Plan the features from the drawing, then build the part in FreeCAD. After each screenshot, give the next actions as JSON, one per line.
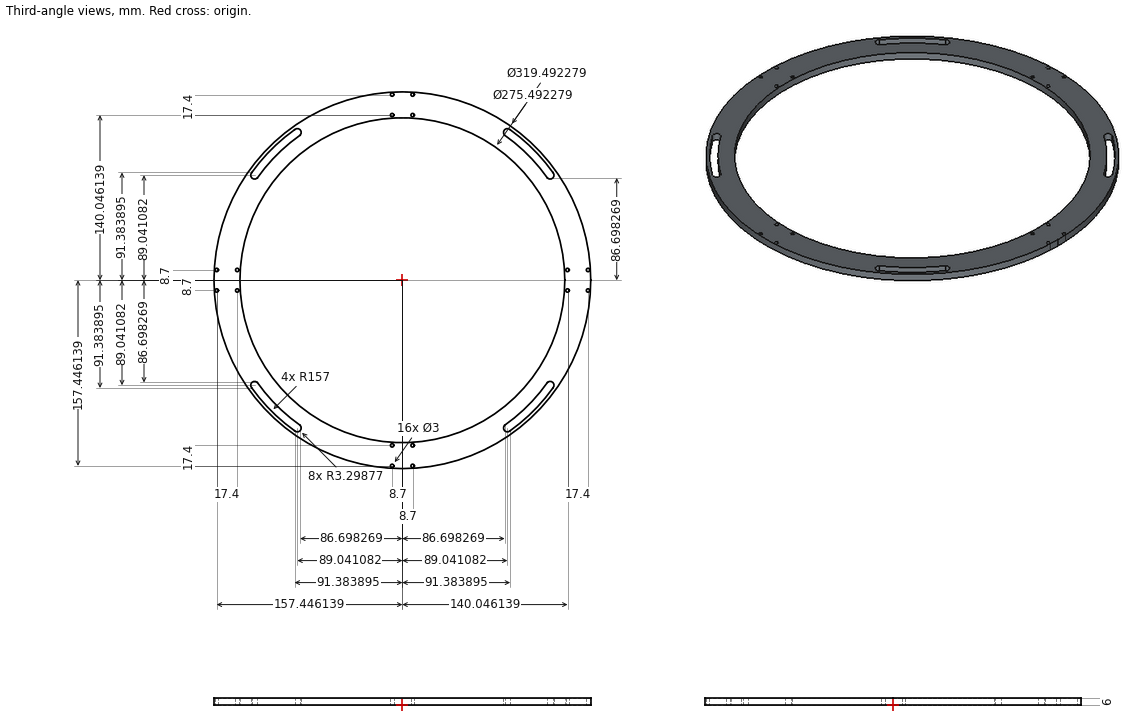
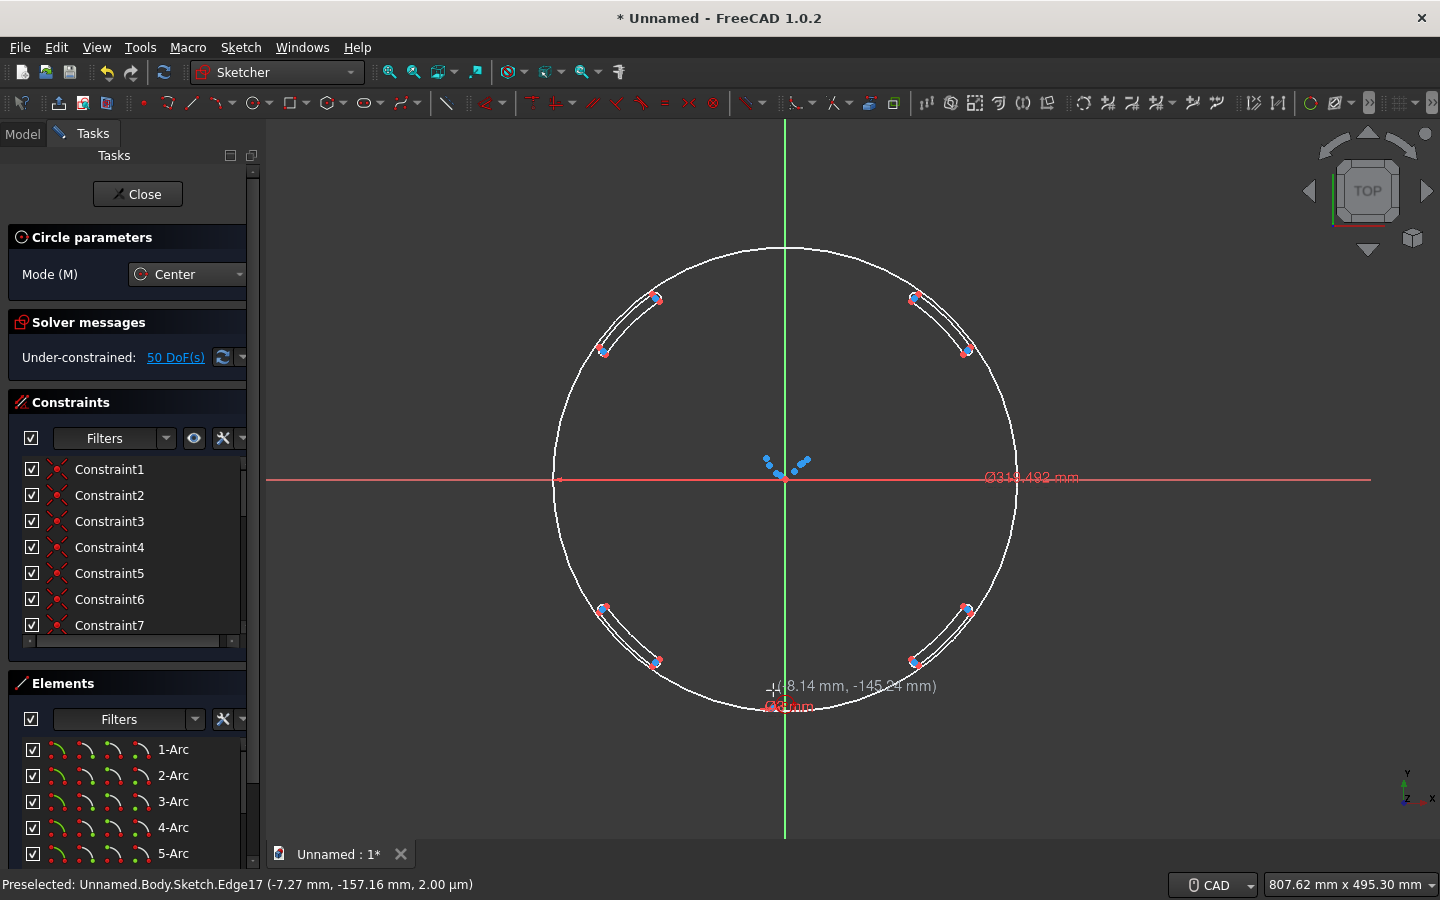
{"action": "scroll", "coordinate": [773, 683], "scroll_direction": "up", "scroll_amount": 2}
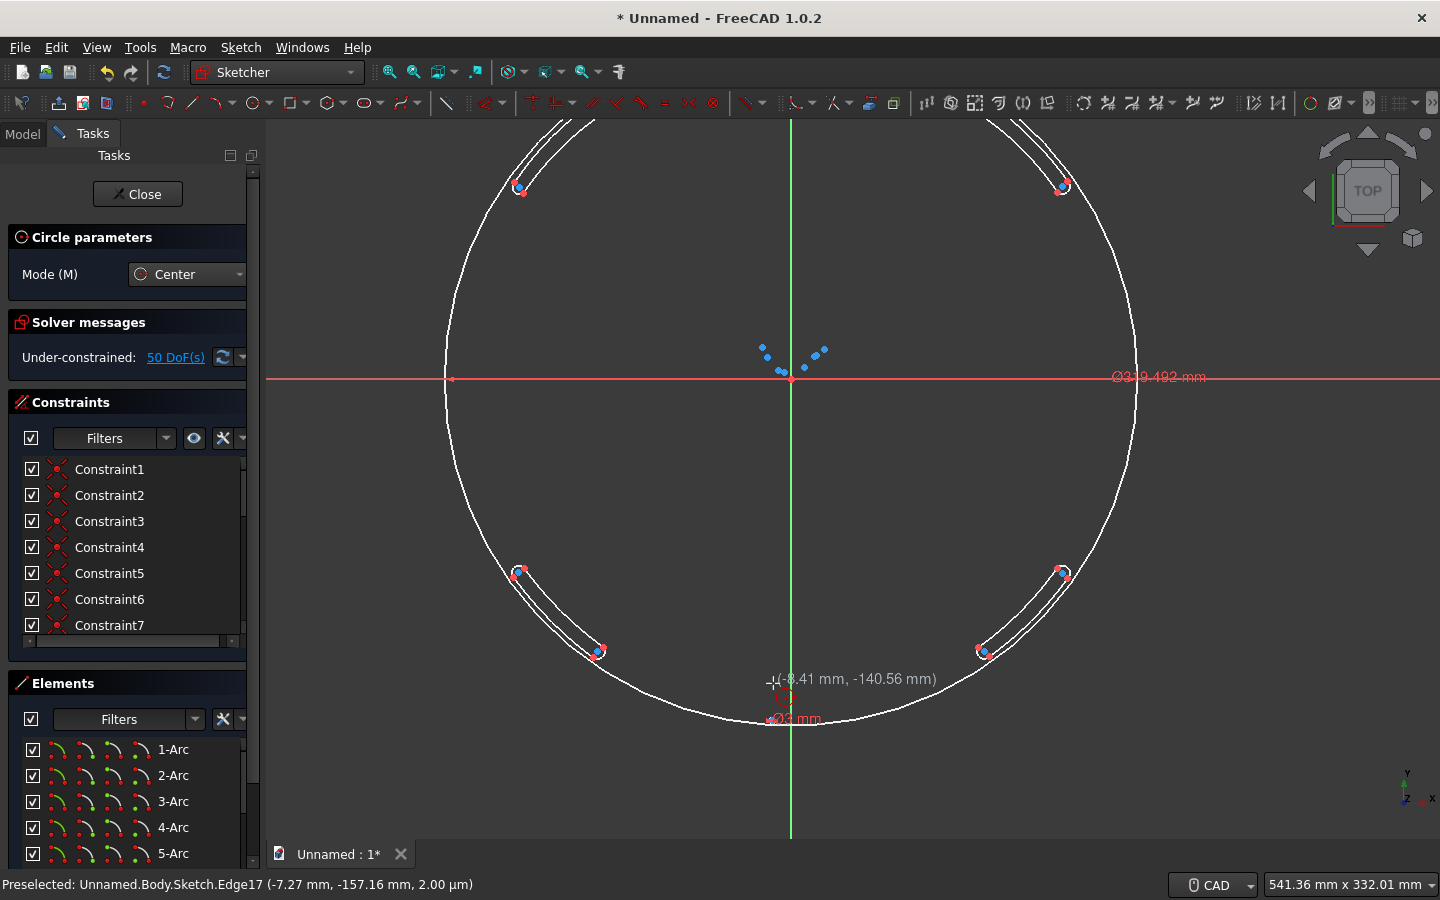
{"action": "left_click", "coordinate": [772, 683]}
{"action": "mouse_move", "coordinate": [774, 681]}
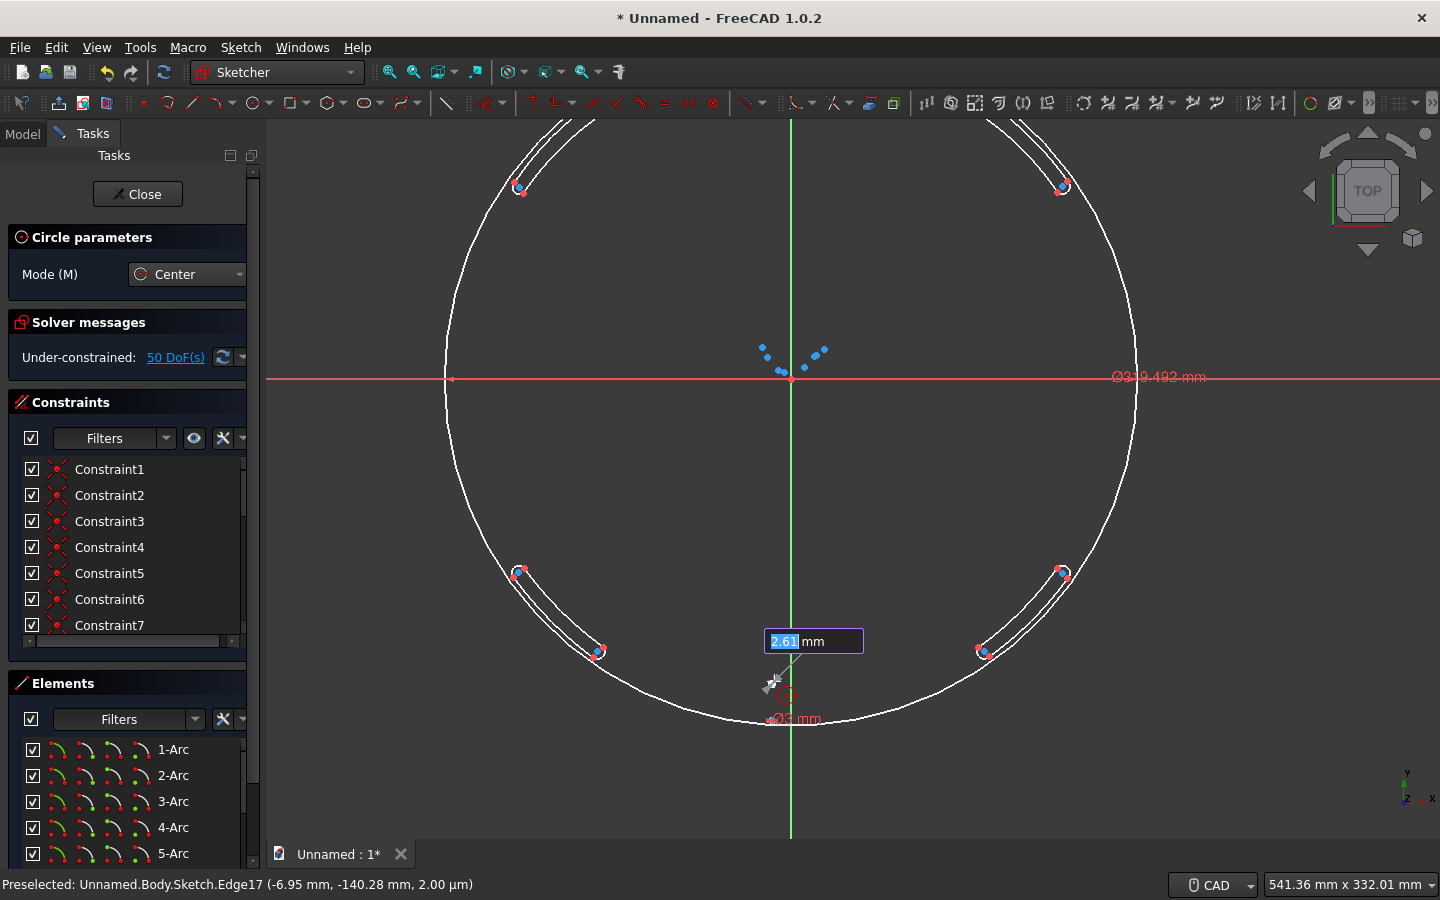
{"action": "type", "text": "3"}
{"action": "key", "text": "Return"}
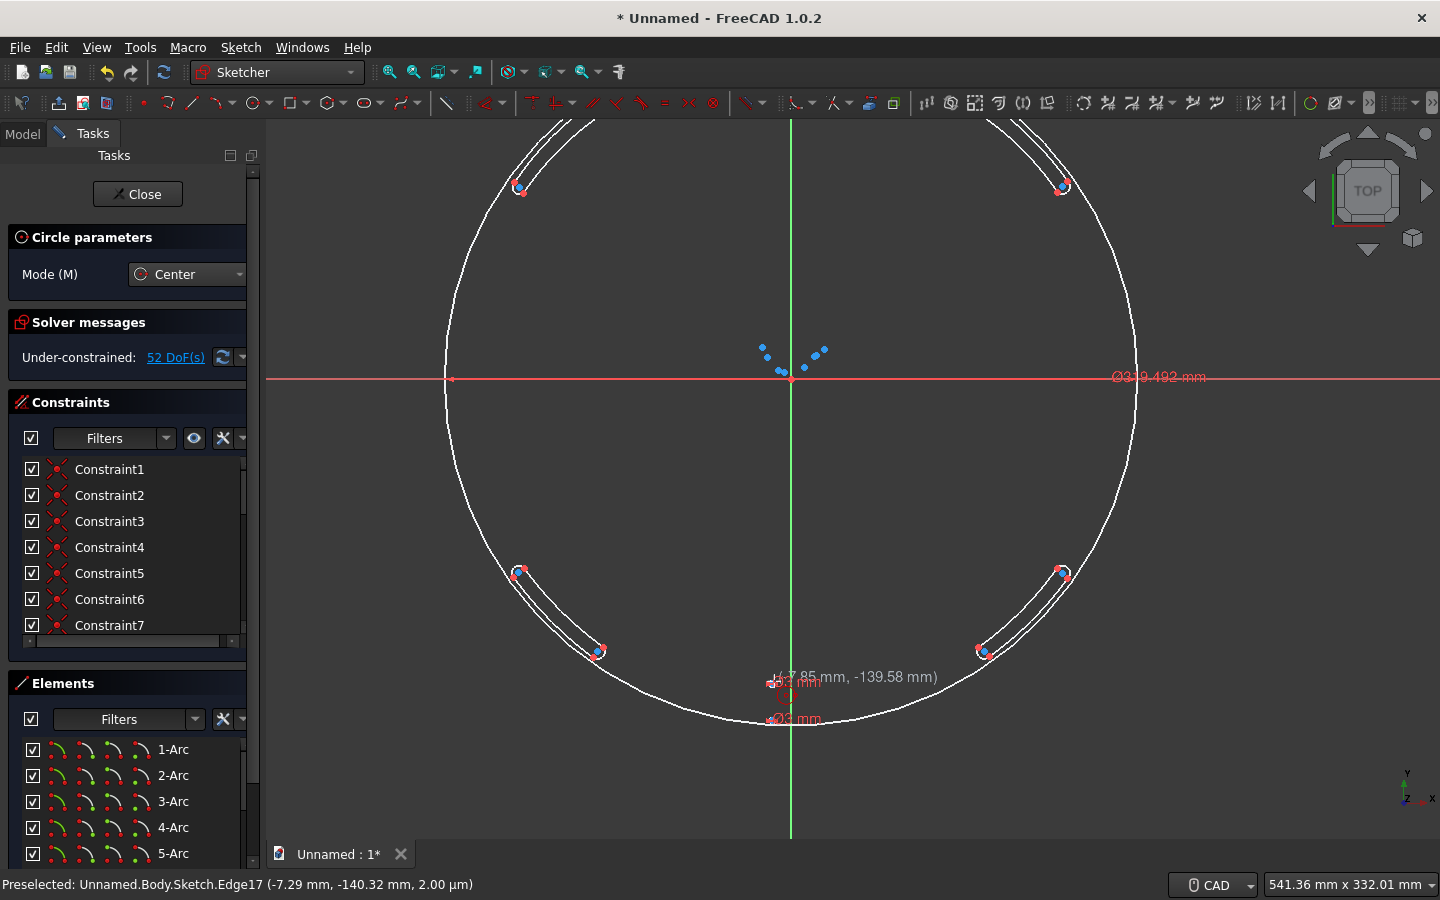
{"action": "scroll", "coordinate": [450, 398], "scroll_direction": "up", "scroll_amount": 10}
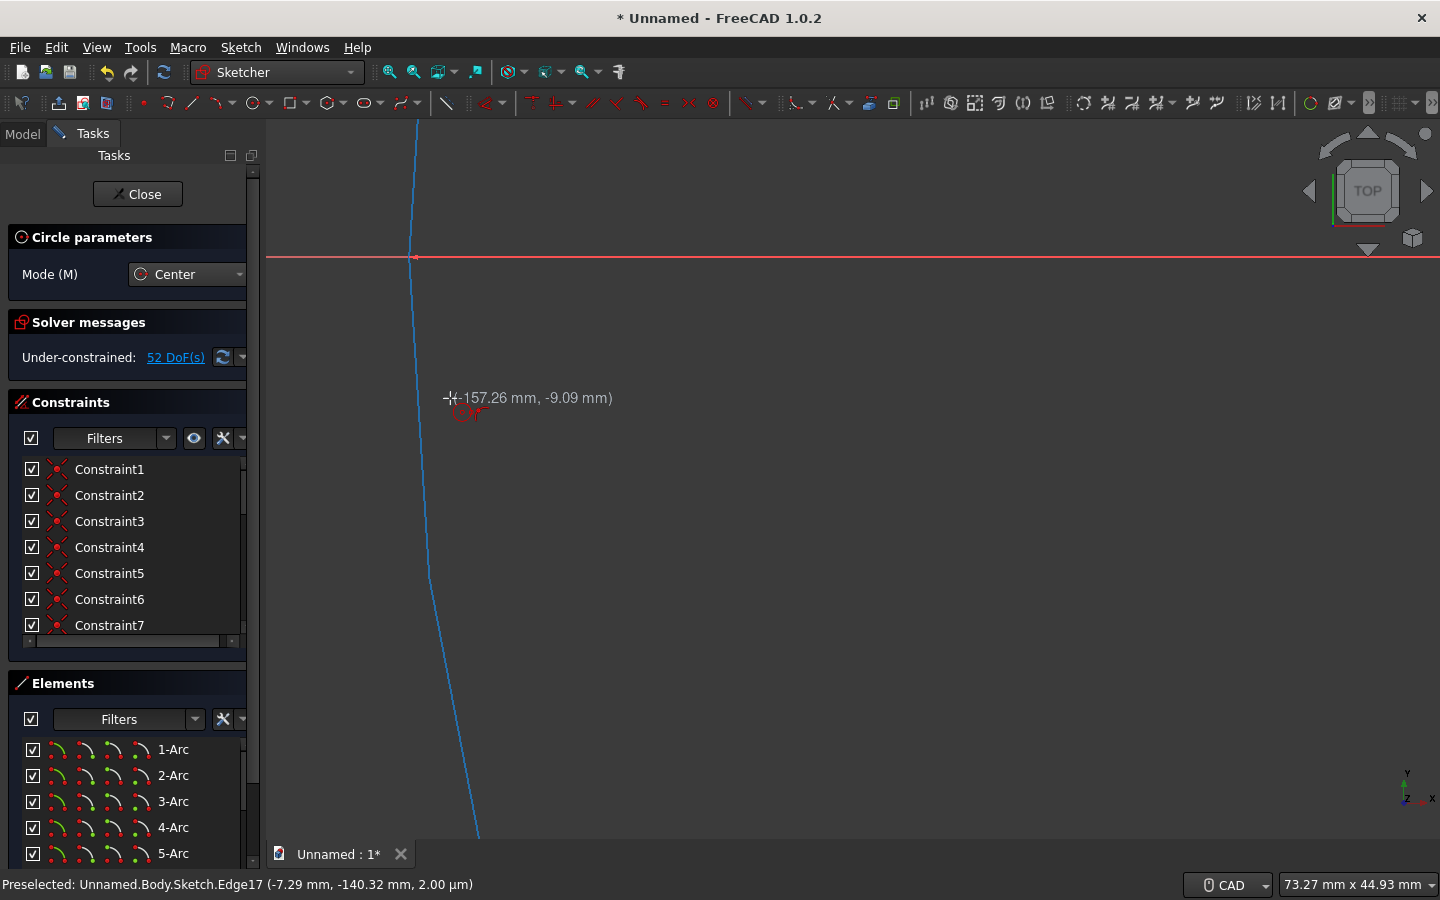
{"action": "left_click", "coordinate": [446, 397]}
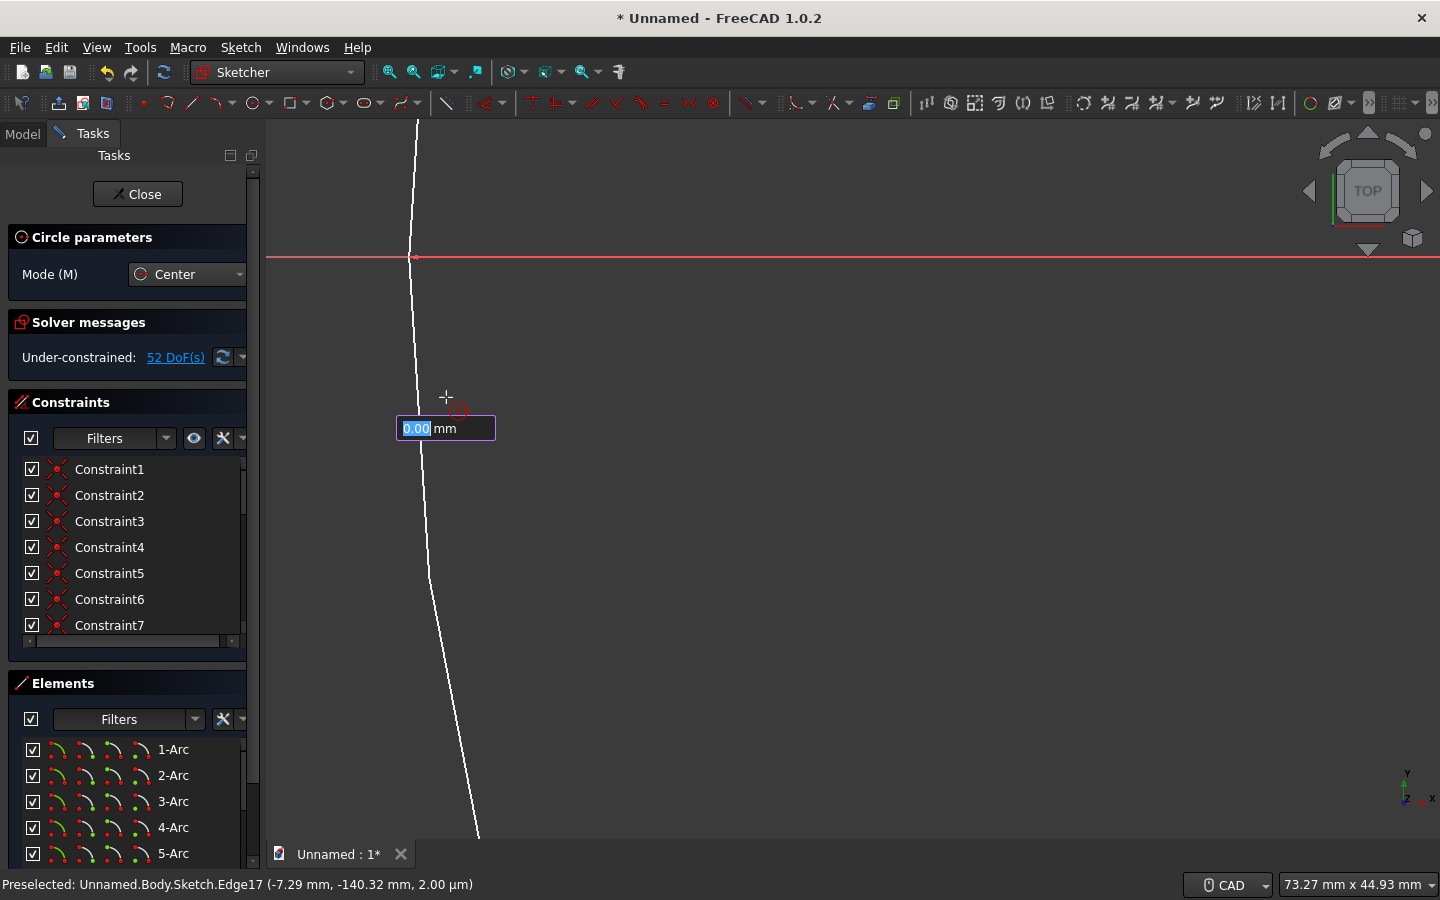
{"action": "scroll", "coordinate": [567, 501], "scroll_direction": "down", "scroll_amount": 12}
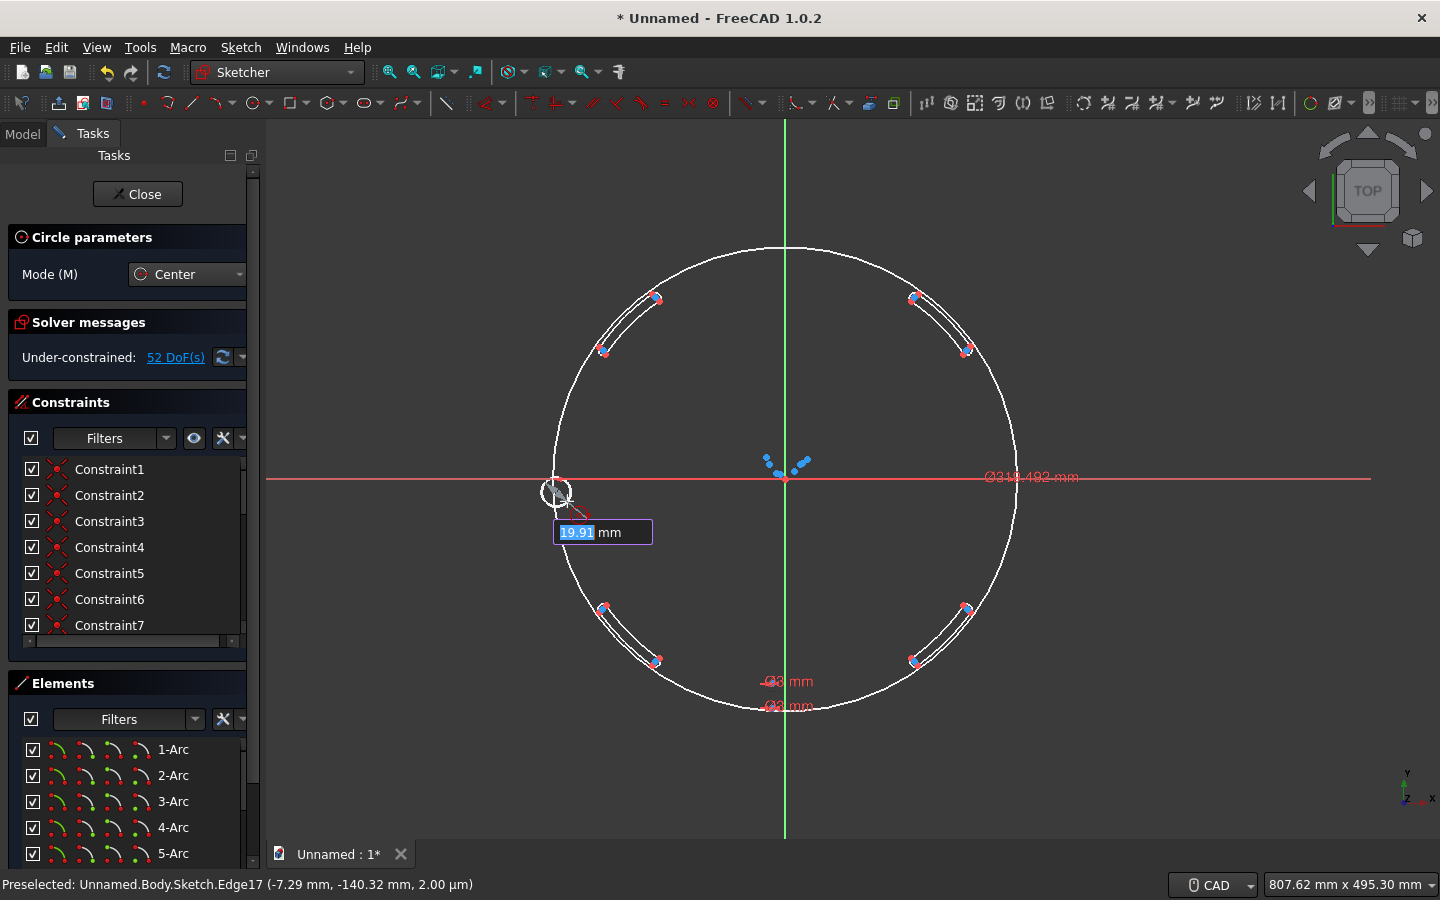
{"action": "scroll", "coordinate": [558, 490], "scroll_direction": "up", "scroll_amount": 7}
{"action": "mouse_move", "coordinate": [556, 490]}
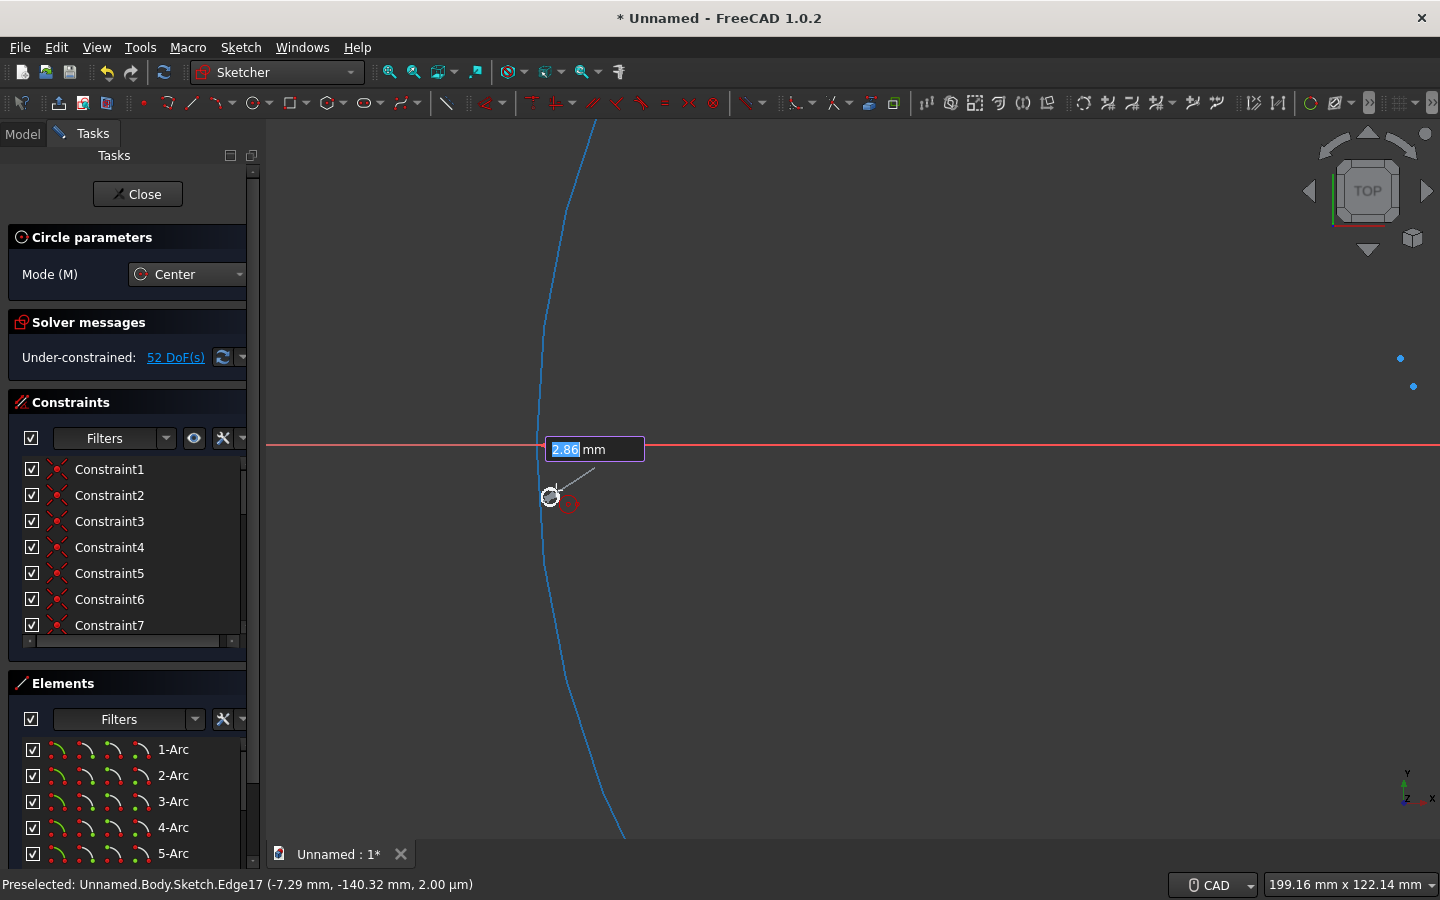
{"action": "type", "text": "3"}
{"action": "key", "text": "Return"}